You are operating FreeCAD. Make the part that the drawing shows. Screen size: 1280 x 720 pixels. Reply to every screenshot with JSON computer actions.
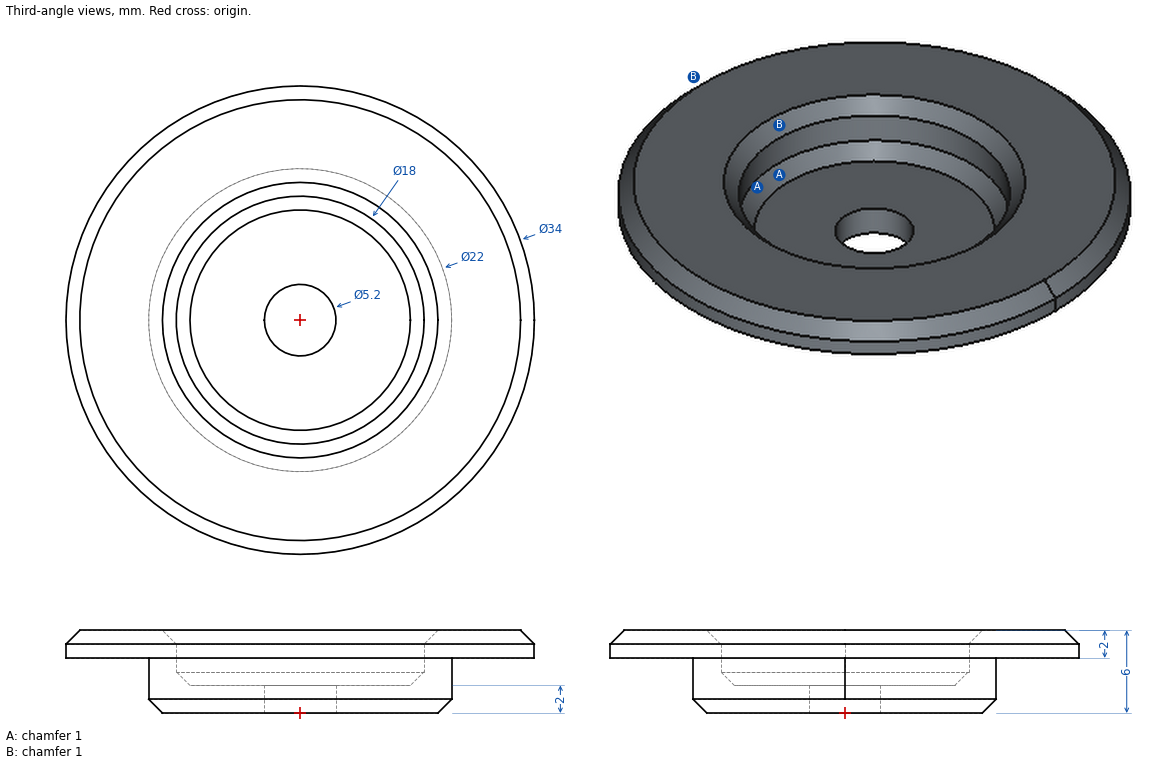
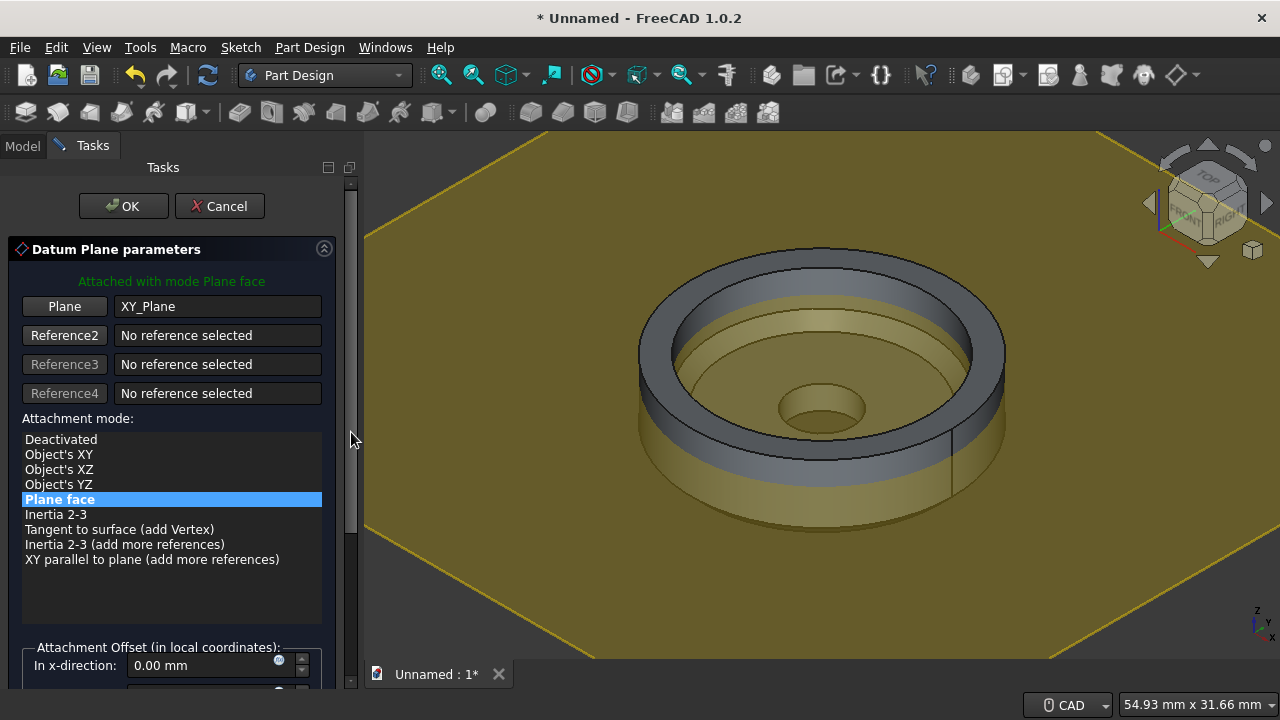
{"action": "left_click", "coordinate": [124, 206]}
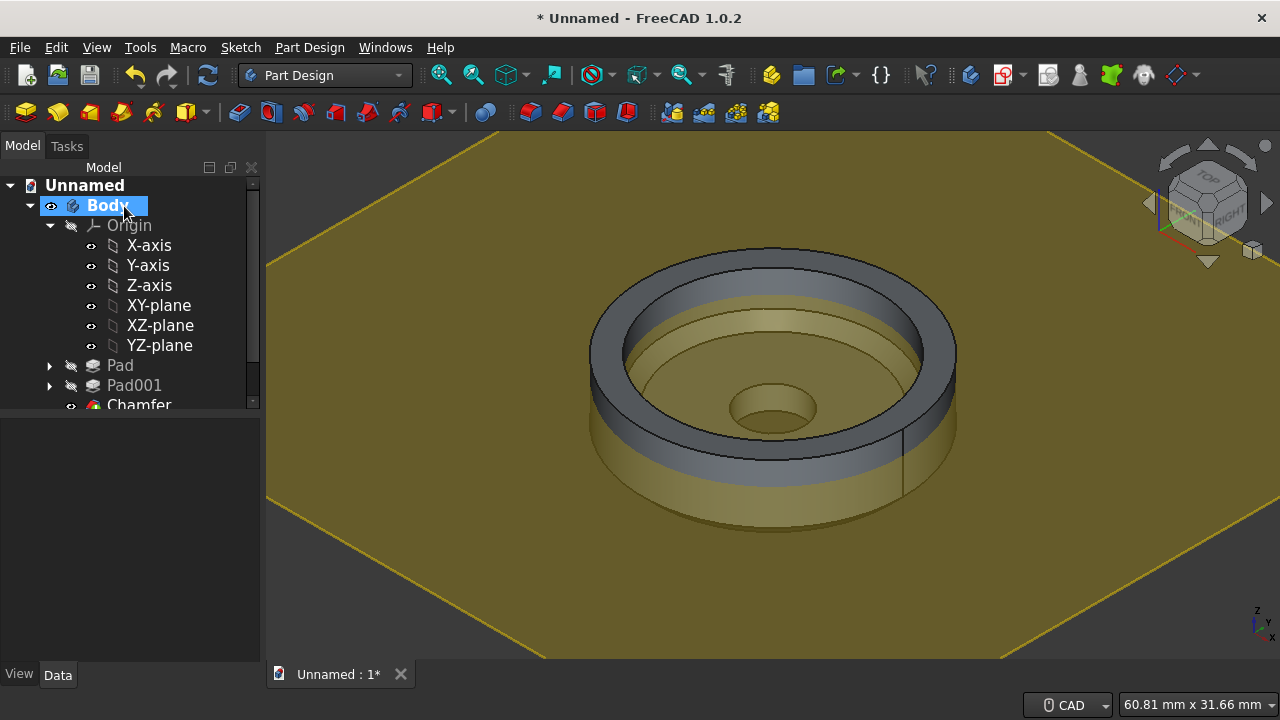
{"action": "scroll", "coordinate": [100, 301], "scroll_direction": "down", "scroll_amount": 3}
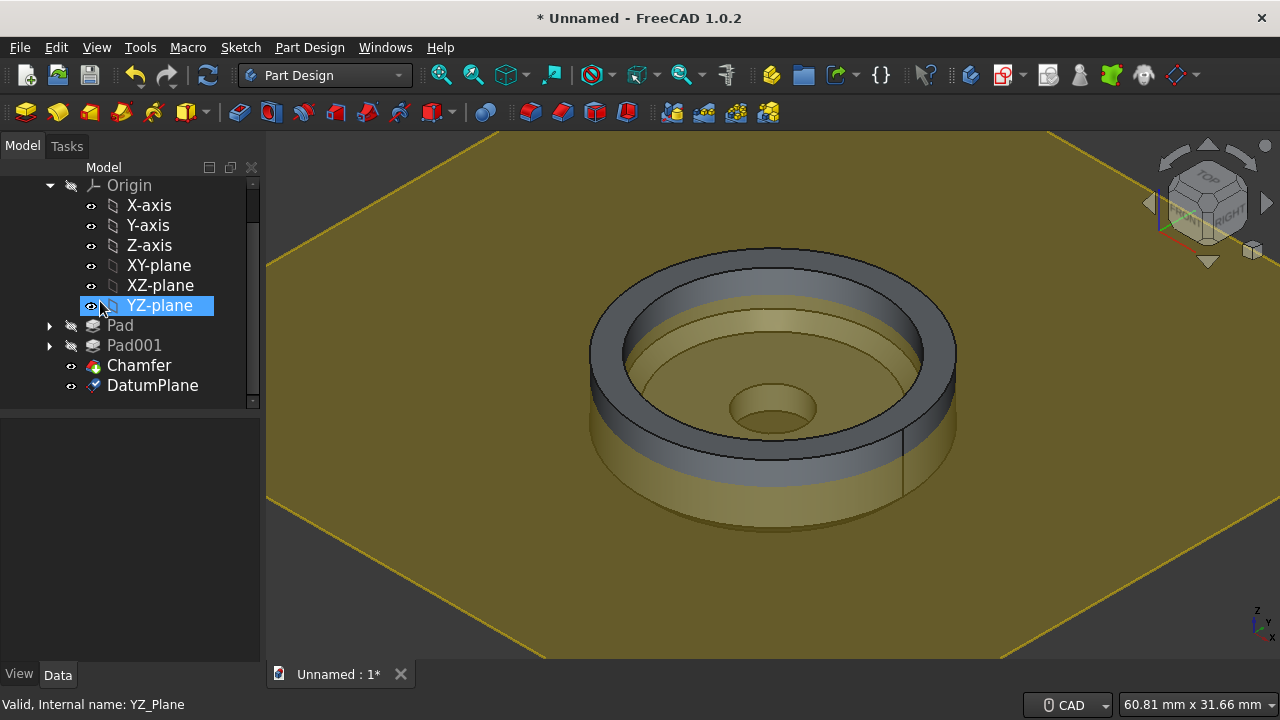
{"action": "left_click", "coordinate": [116, 386]}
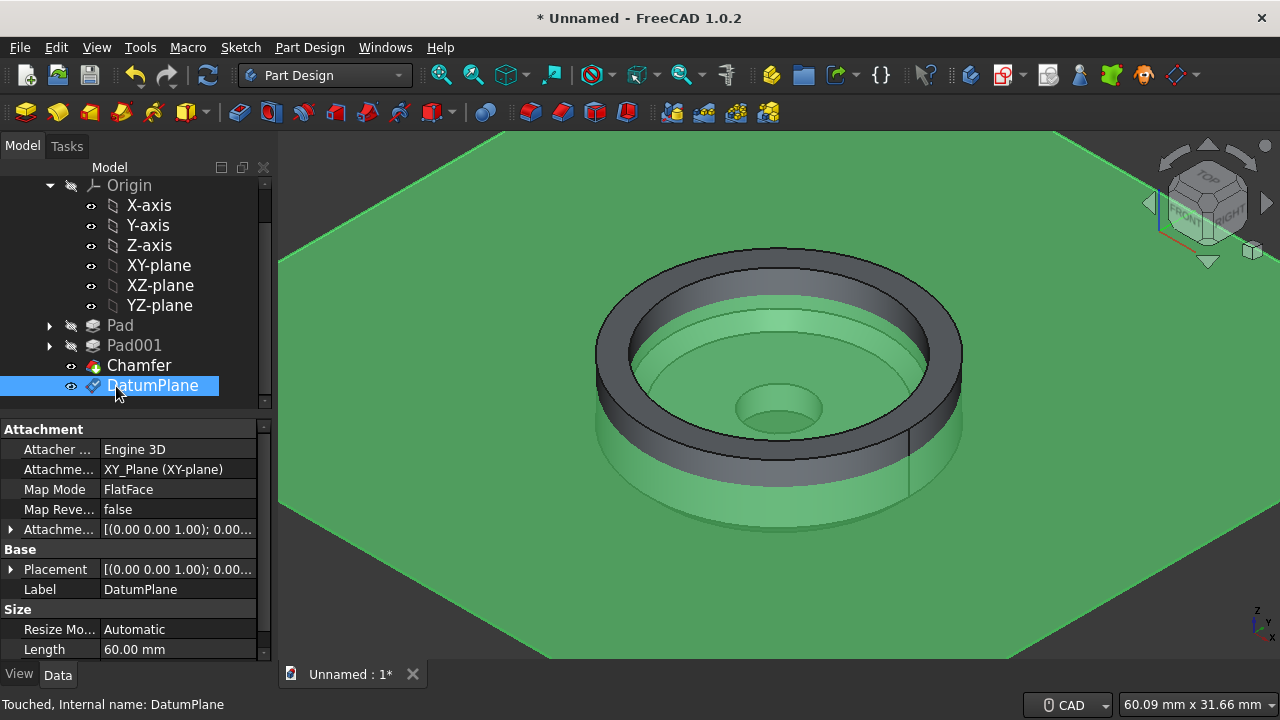
{"action": "left_click", "coordinate": [1004, 76]}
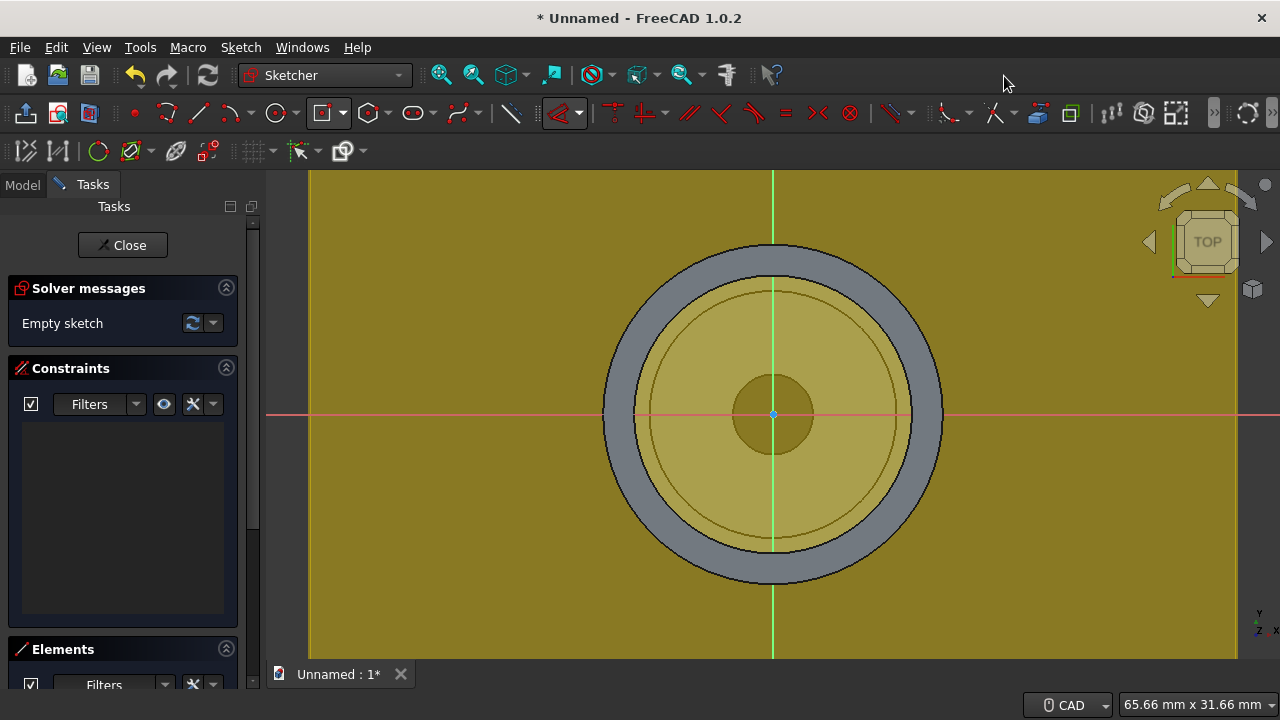
{"action": "left_click", "coordinate": [90, 114]}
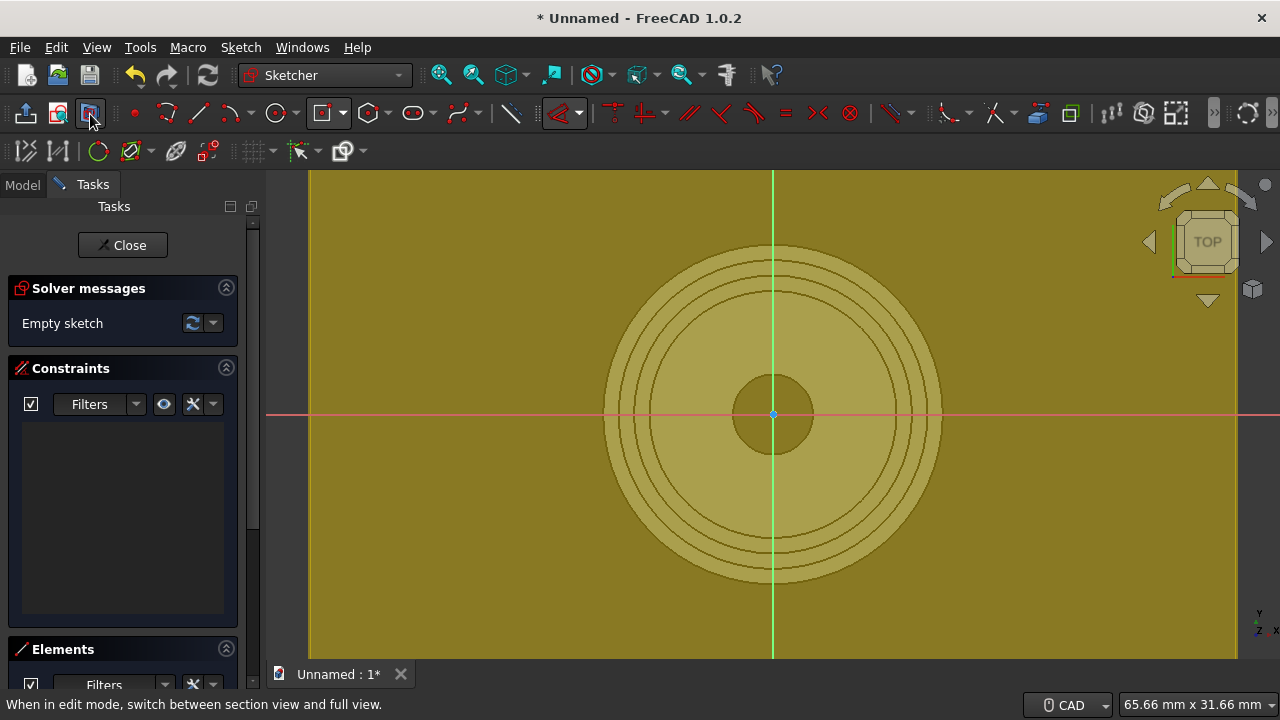
{"action": "scroll", "coordinate": [621, 414], "scroll_direction": "down", "scroll_amount": 3}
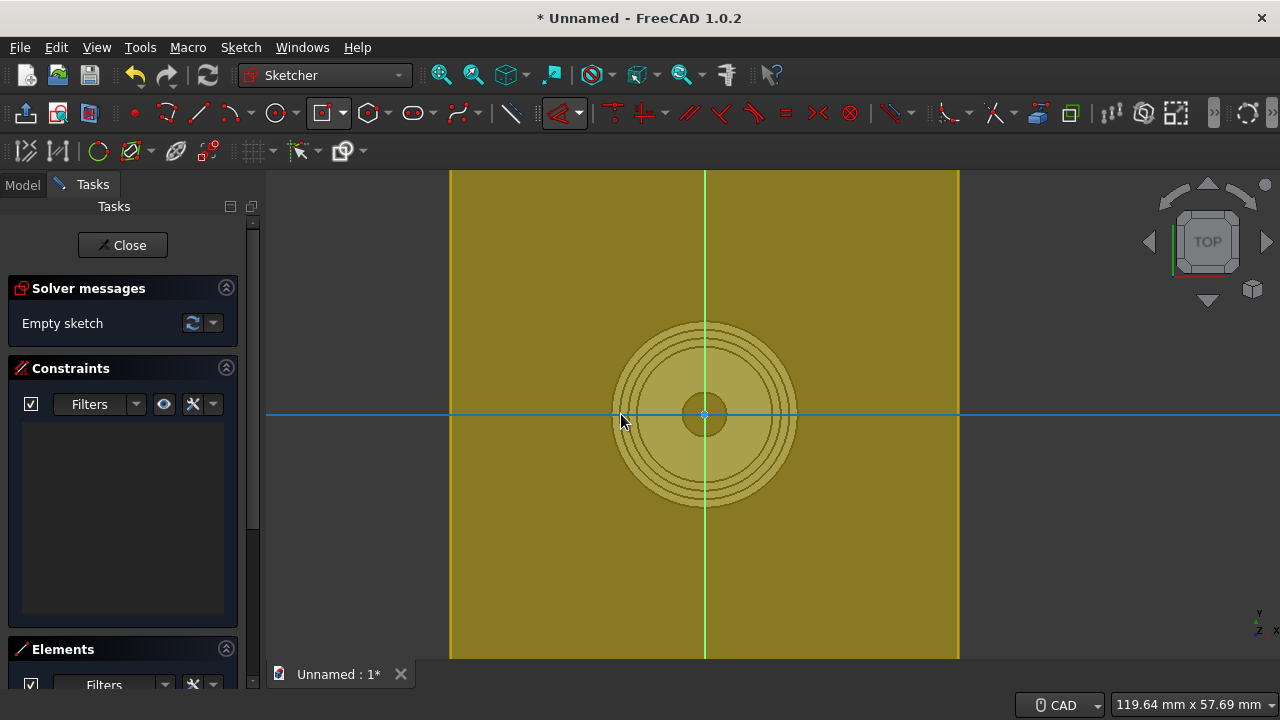
{"action": "left_click", "coordinate": [276, 114]}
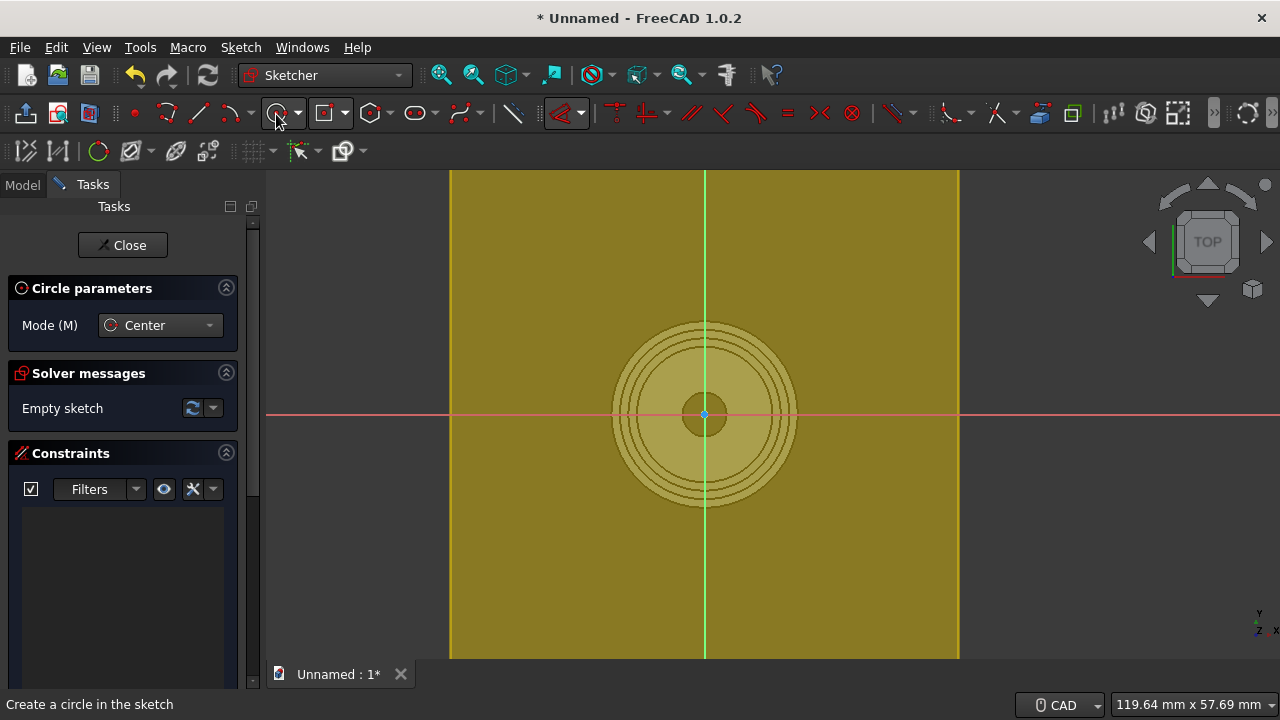
{"action": "left_click", "coordinate": [705, 414]}
{"action": "mouse_move", "coordinate": [806, 313]}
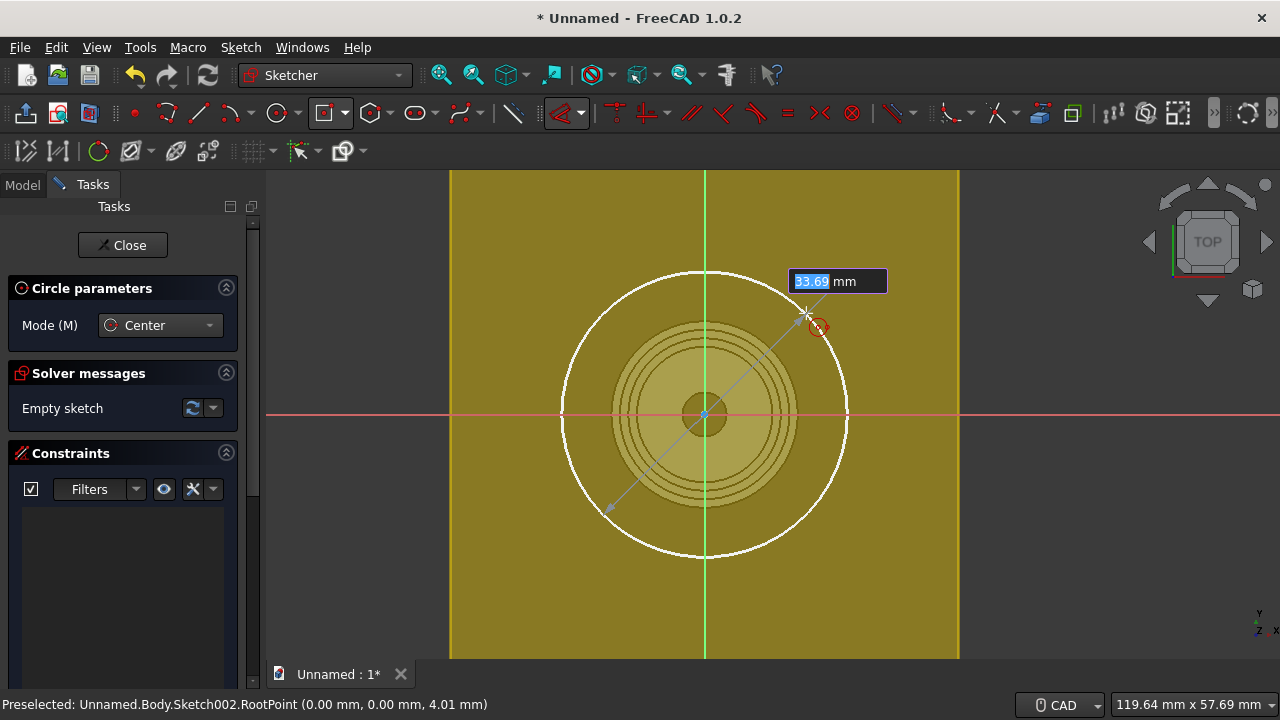
{"action": "type", "text": "34"}
{"action": "key", "text": "Return"}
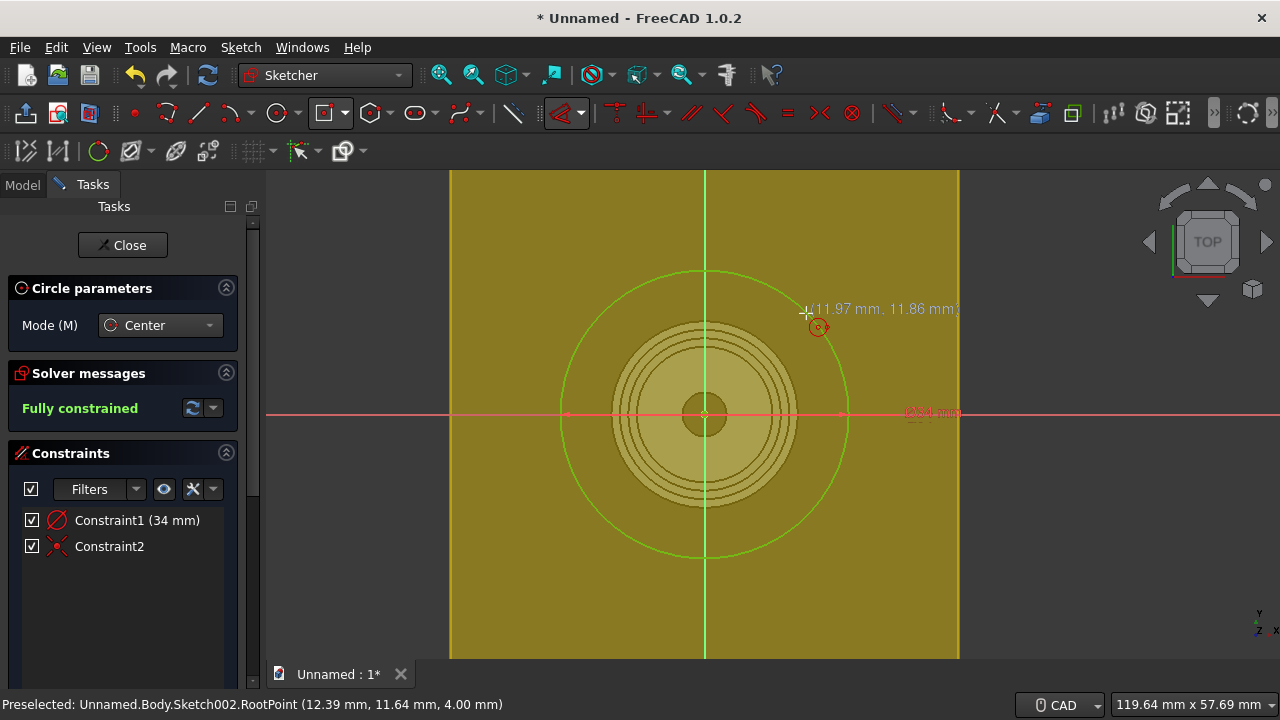
{"action": "left_click", "coordinate": [705, 414]}
{"action": "mouse_move", "coordinate": [759, 361]}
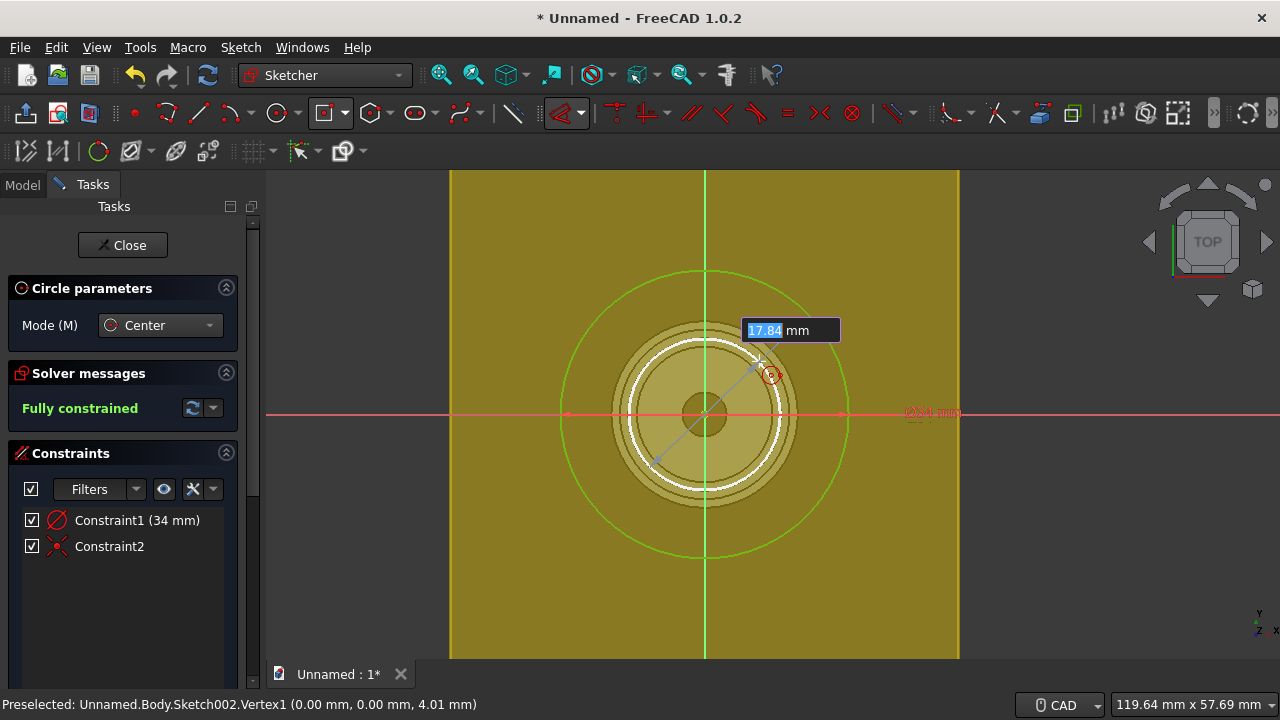
{"action": "type", "text": "18"}
{"action": "key", "text": "Return"}
{"action": "key", "text": "Escape"}